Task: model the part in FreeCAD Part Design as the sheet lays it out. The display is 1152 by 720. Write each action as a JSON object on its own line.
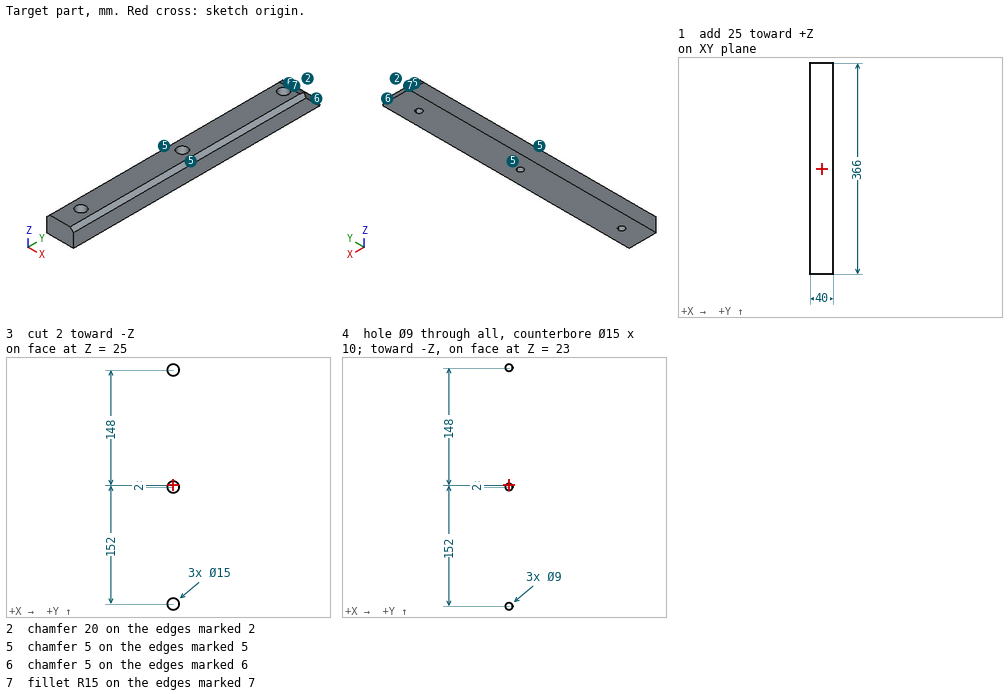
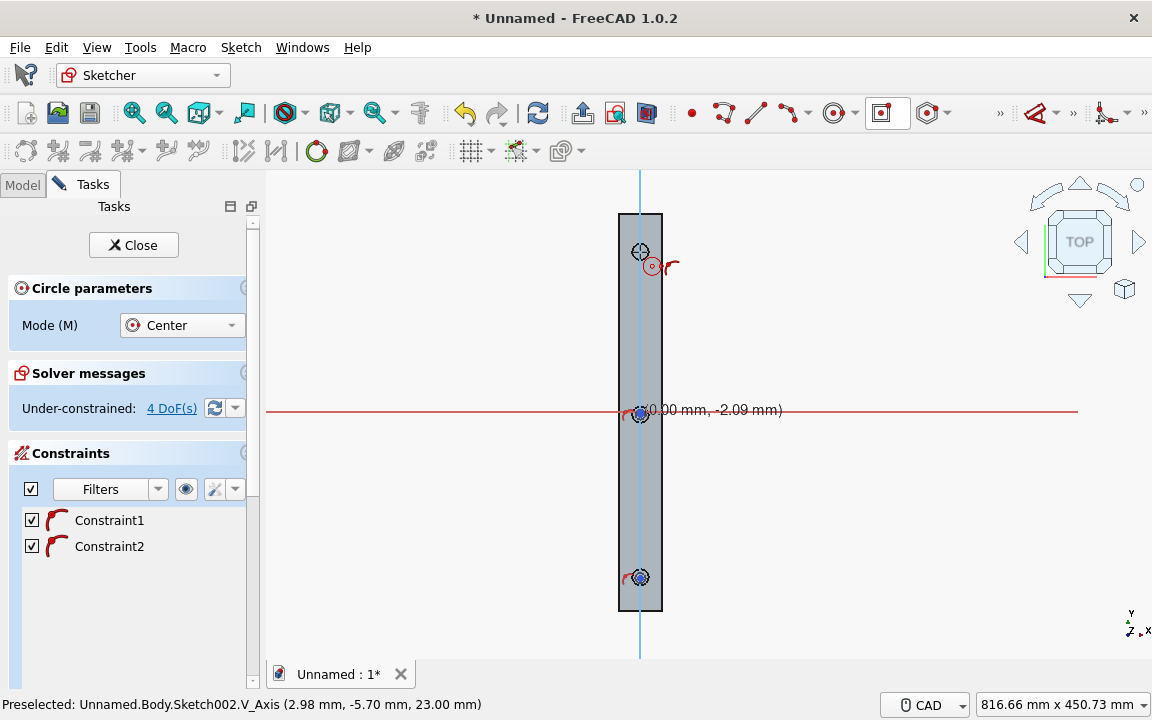
{"action": "left_click", "coordinate": [640, 252]}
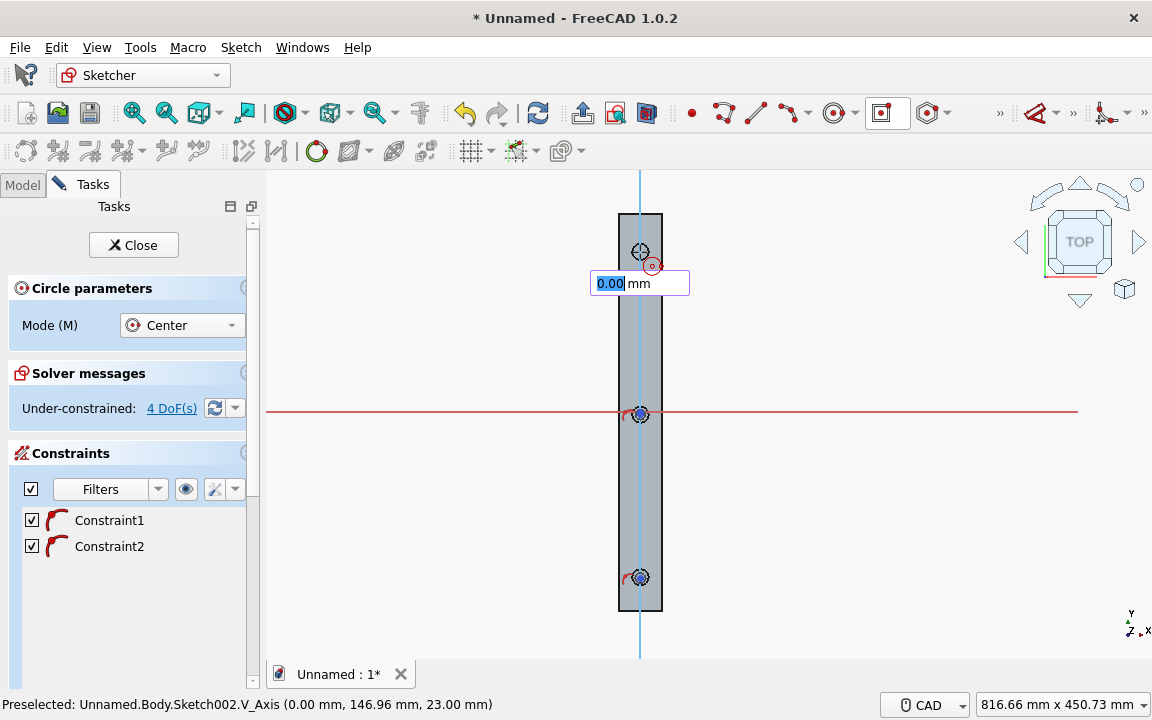
{"action": "scroll", "coordinate": [645, 250], "scroll_direction": "up", "scroll_amount": 7}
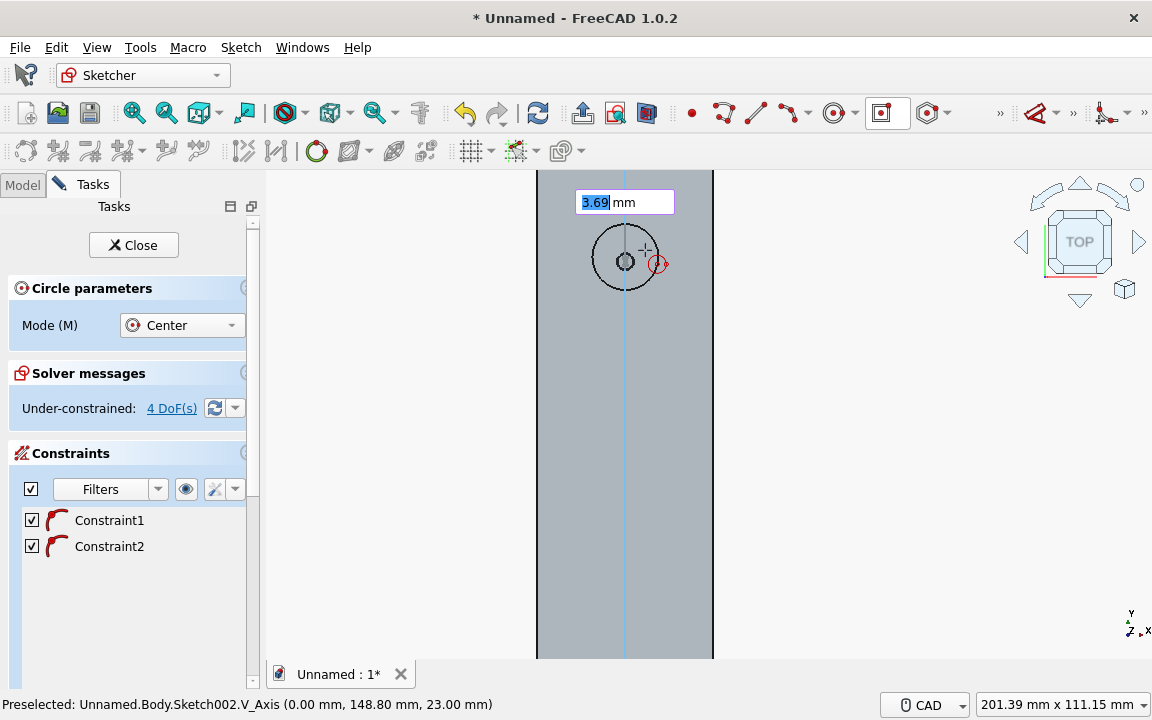
{"action": "left_click", "coordinate": [644, 250]}
{"action": "key", "text": "Escape"}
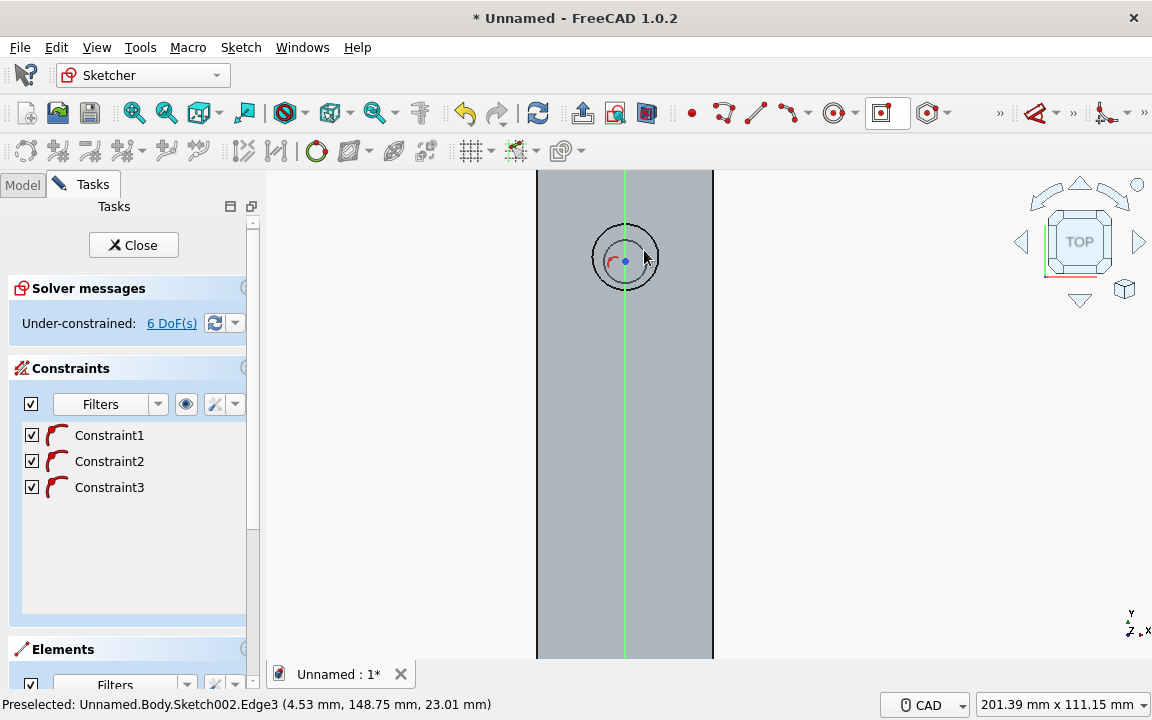
{"action": "scroll", "coordinate": [645, 250], "scroll_direction": "down", "scroll_amount": 7}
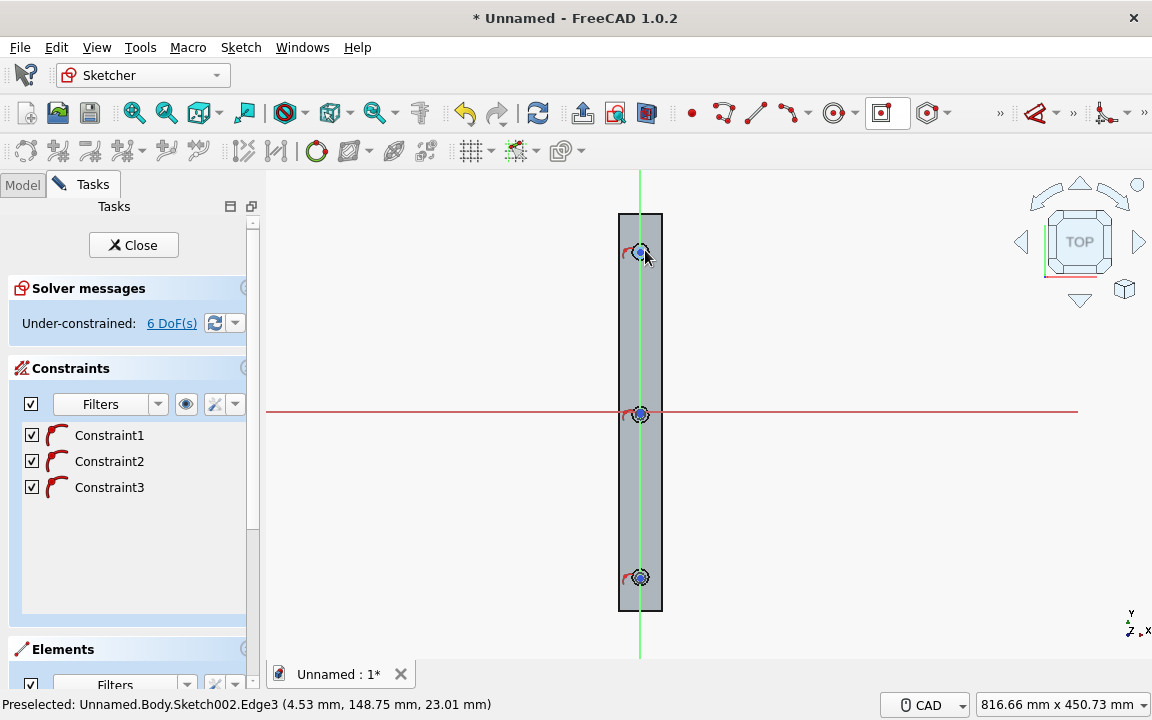
{"action": "scroll", "coordinate": [644, 575], "scroll_direction": "up", "scroll_amount": 7}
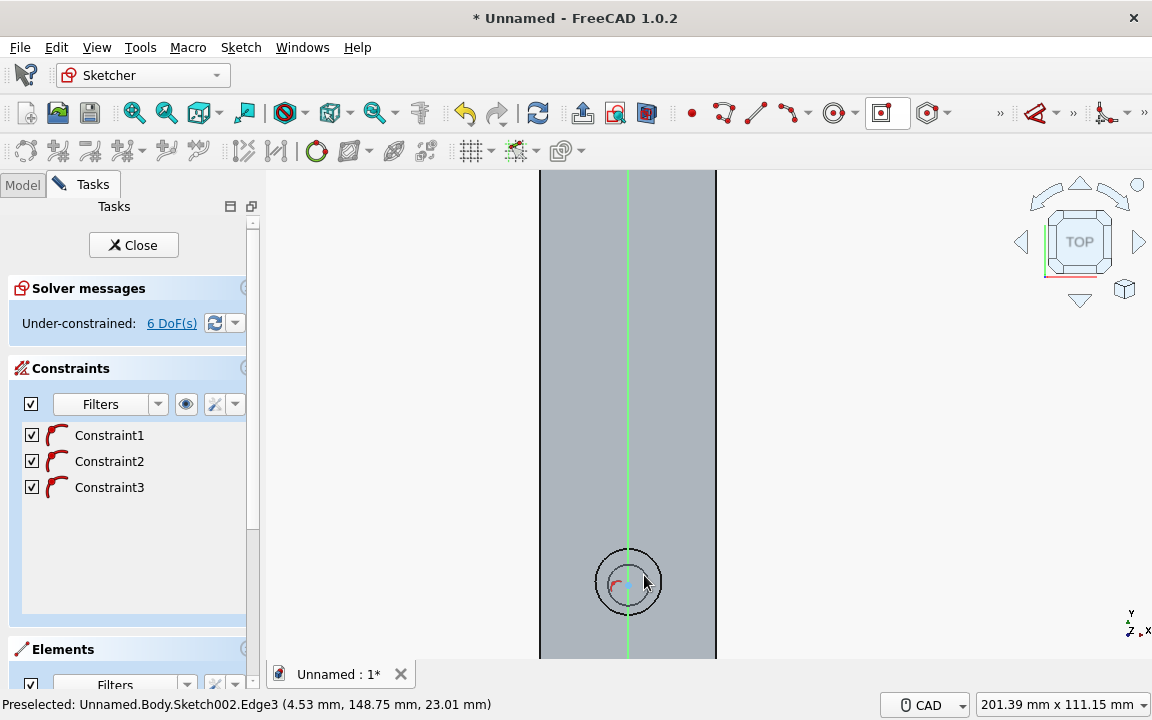
{"action": "left_click", "coordinate": [643, 571]}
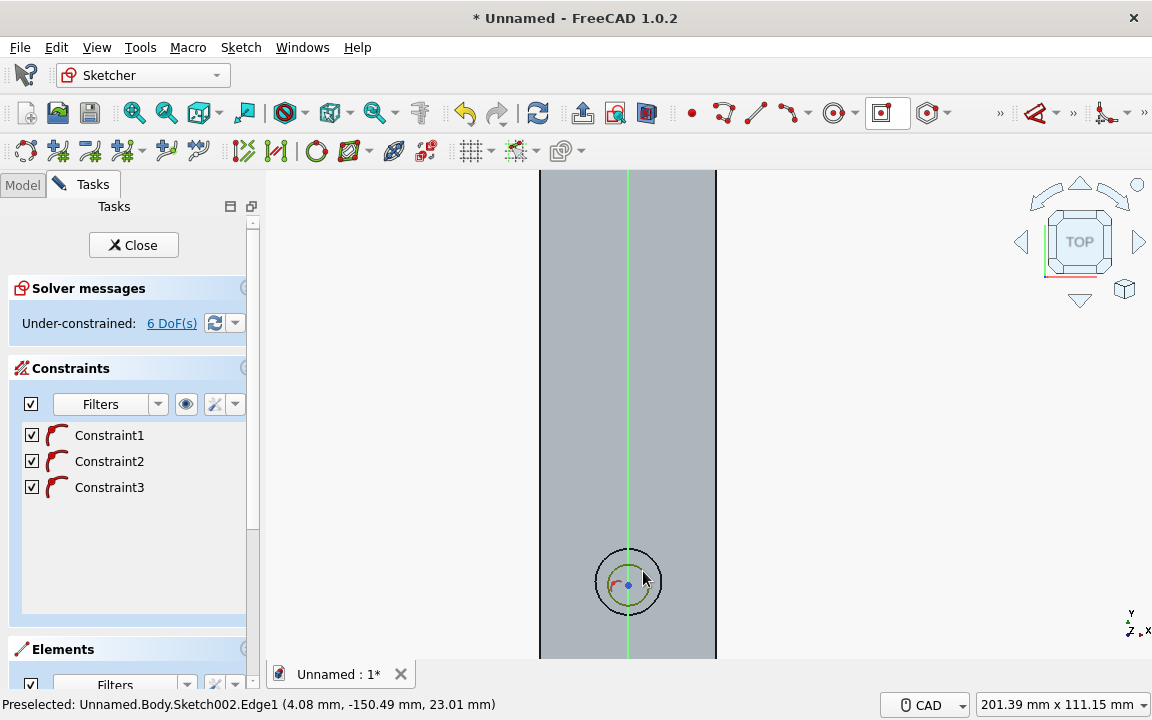
{"action": "scroll", "coordinate": [644, 576], "scroll_direction": "down", "scroll_amount": 7}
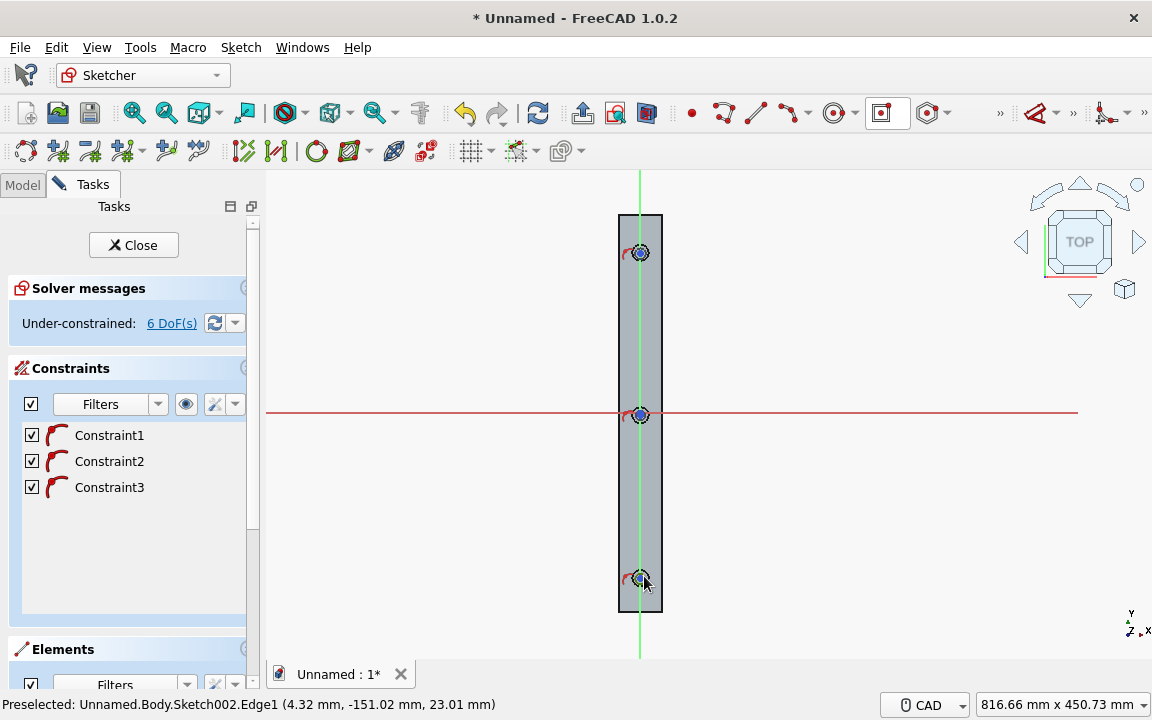
{"action": "scroll", "coordinate": [637, 419], "scroll_direction": "up", "scroll_amount": 7}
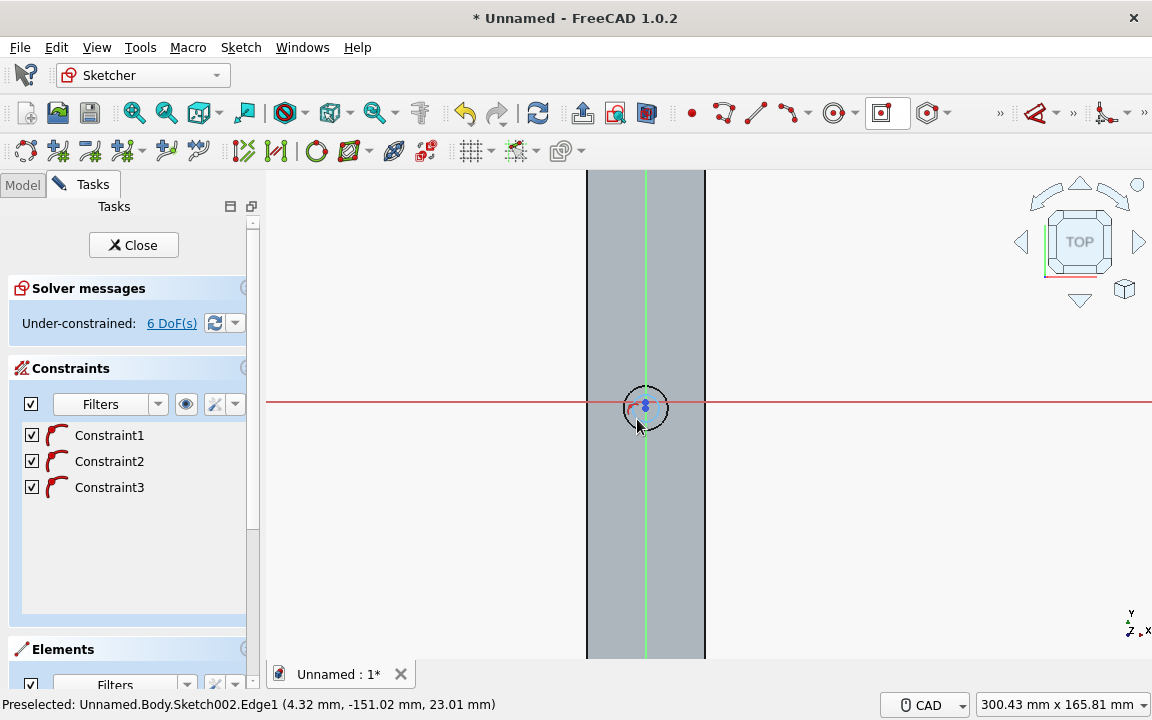
{"action": "left_click", "coordinate": [636, 417]}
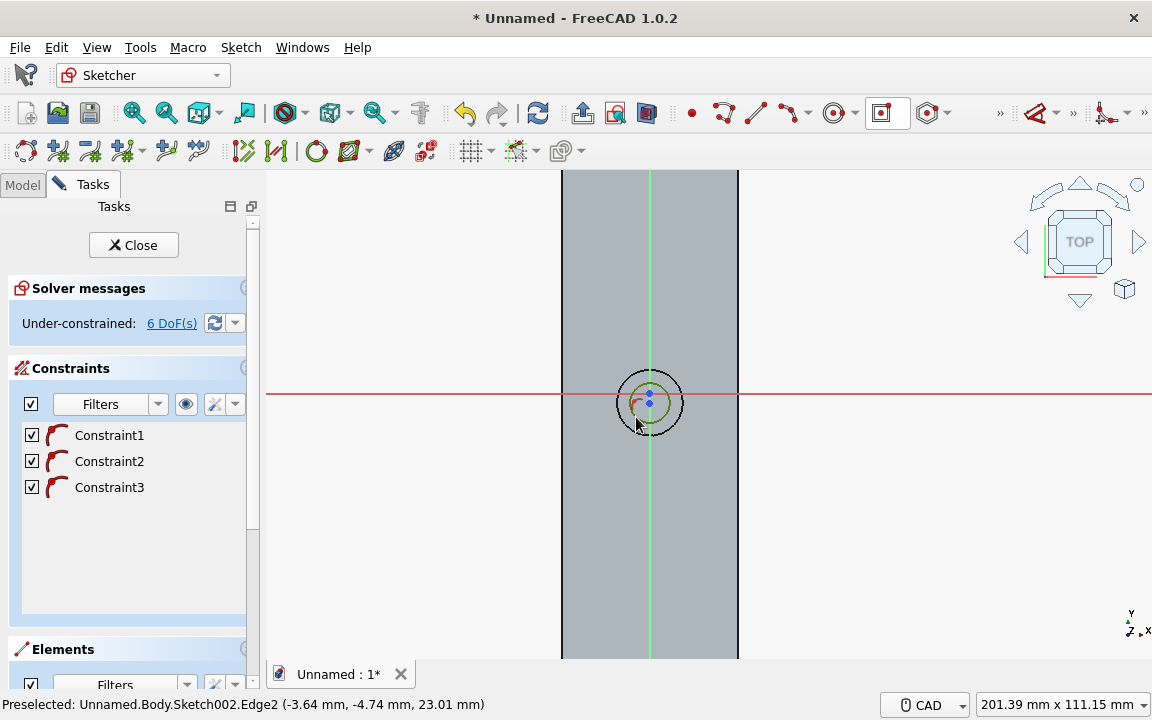
{"action": "scroll", "coordinate": [637, 418], "scroll_direction": "down", "scroll_amount": 7}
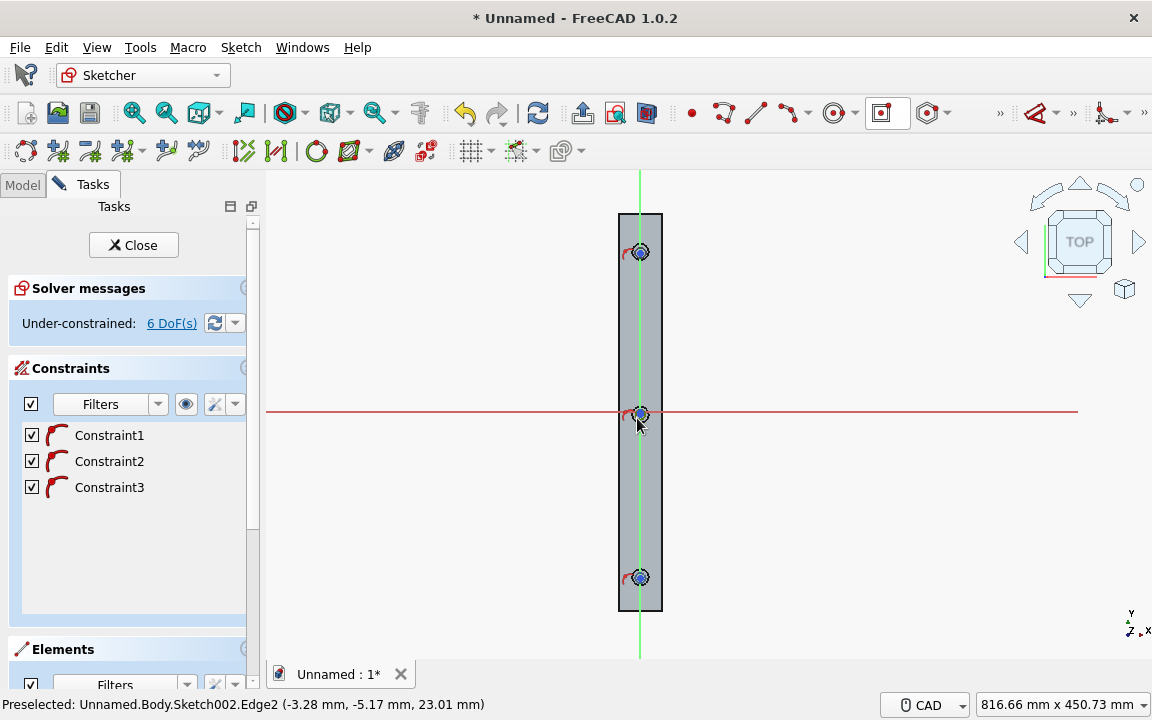
{"action": "scroll", "coordinate": [644, 249], "scroll_direction": "up", "scroll_amount": 7}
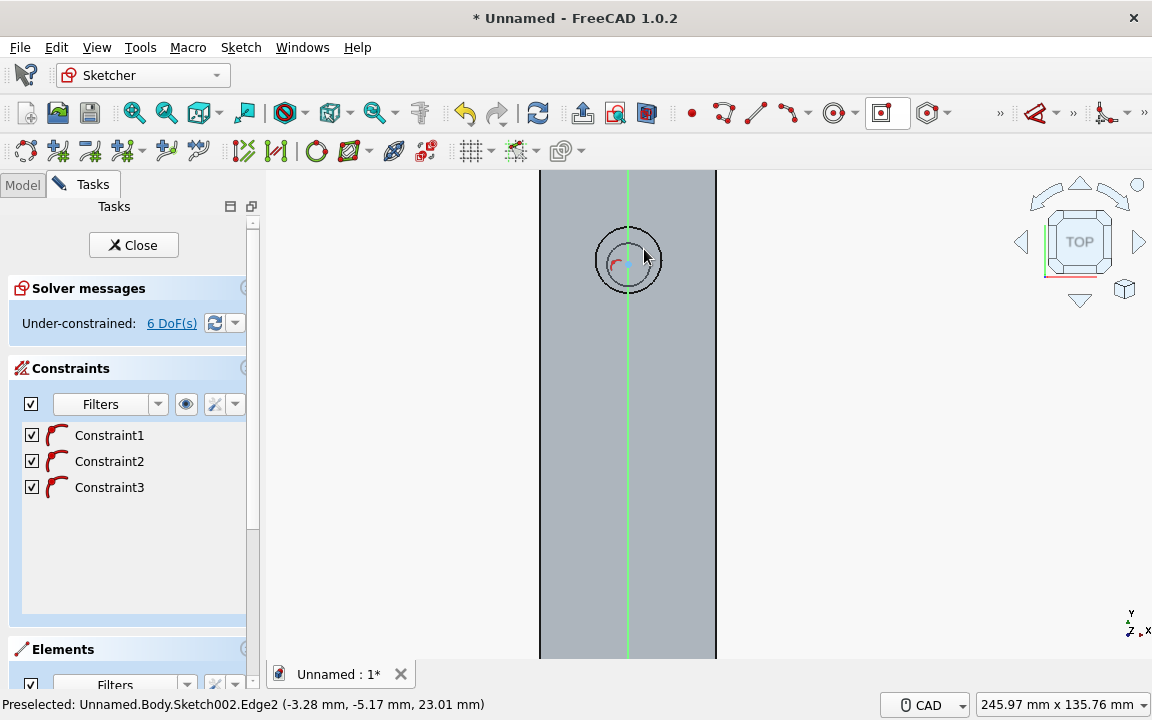
{"action": "left_click", "coordinate": [644, 250]}